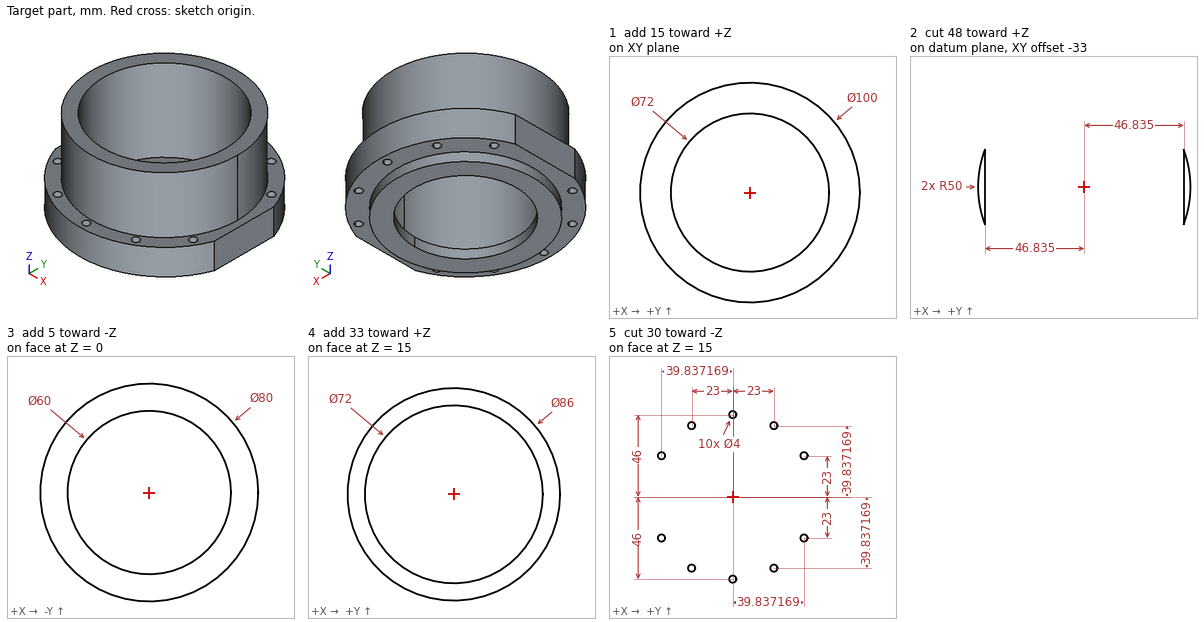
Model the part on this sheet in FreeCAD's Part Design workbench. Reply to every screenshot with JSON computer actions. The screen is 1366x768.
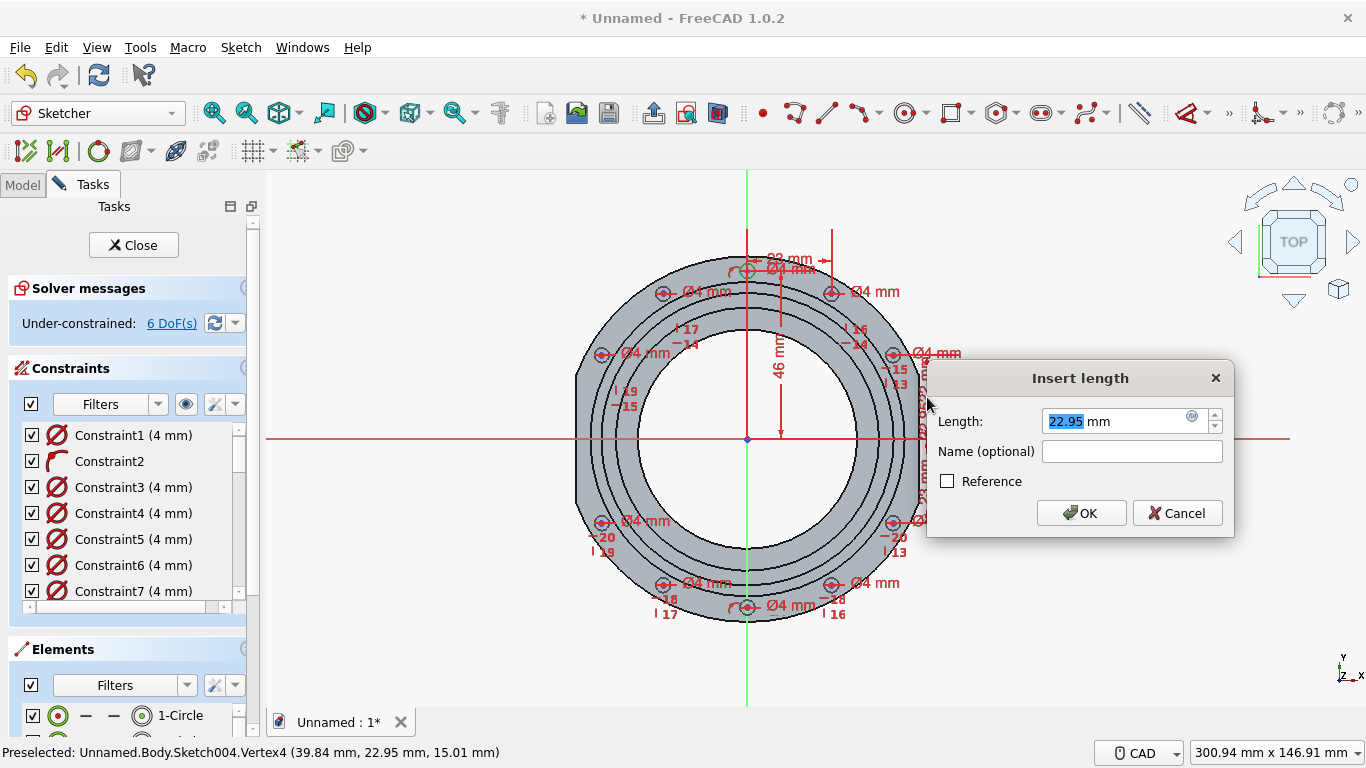
{"action": "type", "text": "23"}
{"action": "key", "text": "Return"}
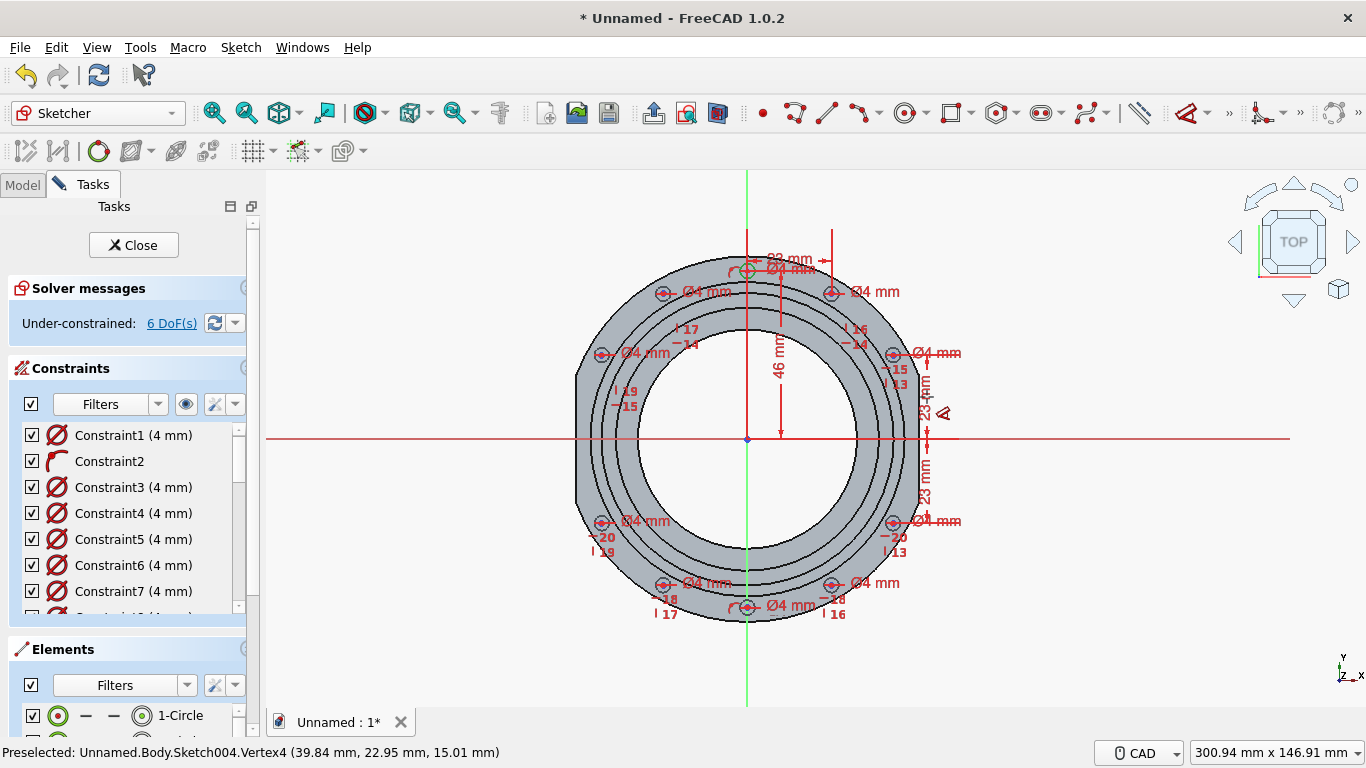
{"action": "left_click", "coordinate": [663, 294]}
{"action": "left_click", "coordinate": [705, 260]}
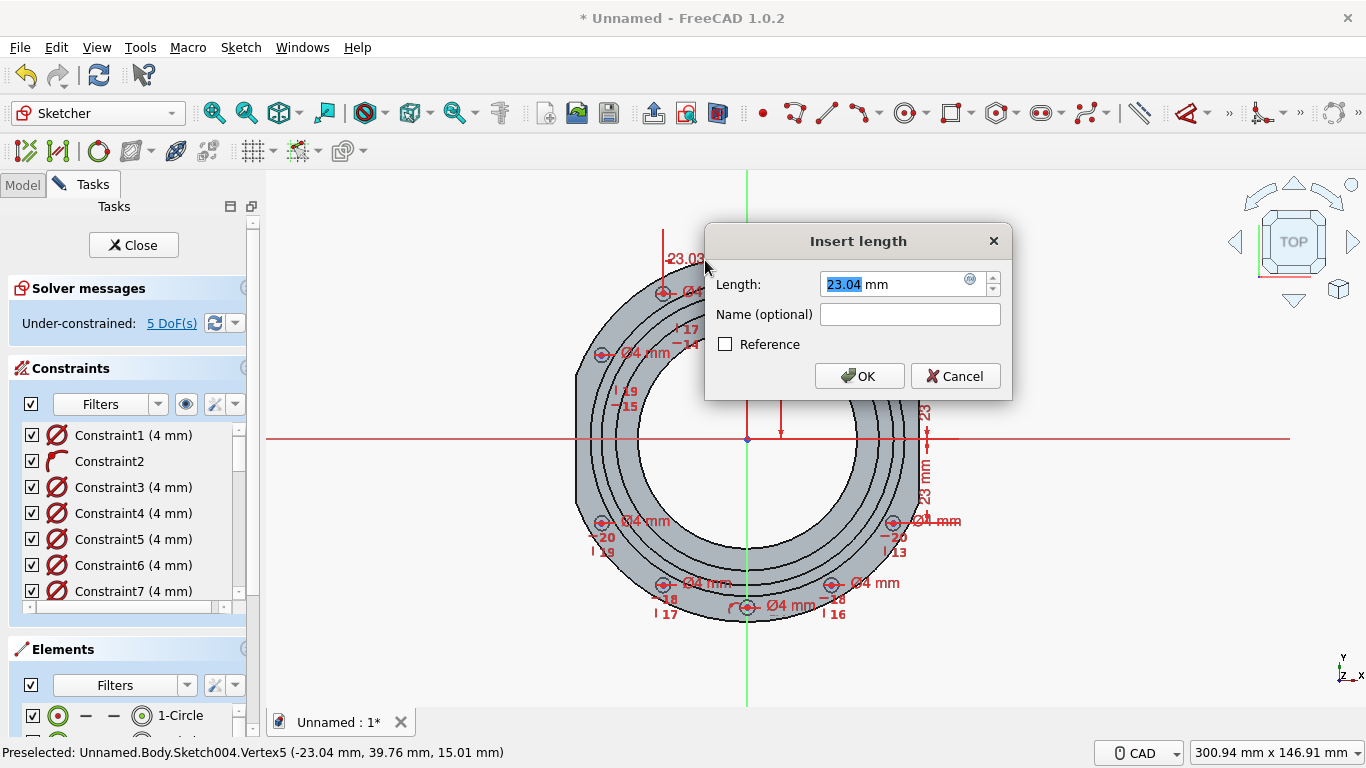
{"action": "type", "text": "23"}
{"action": "key", "text": "Return"}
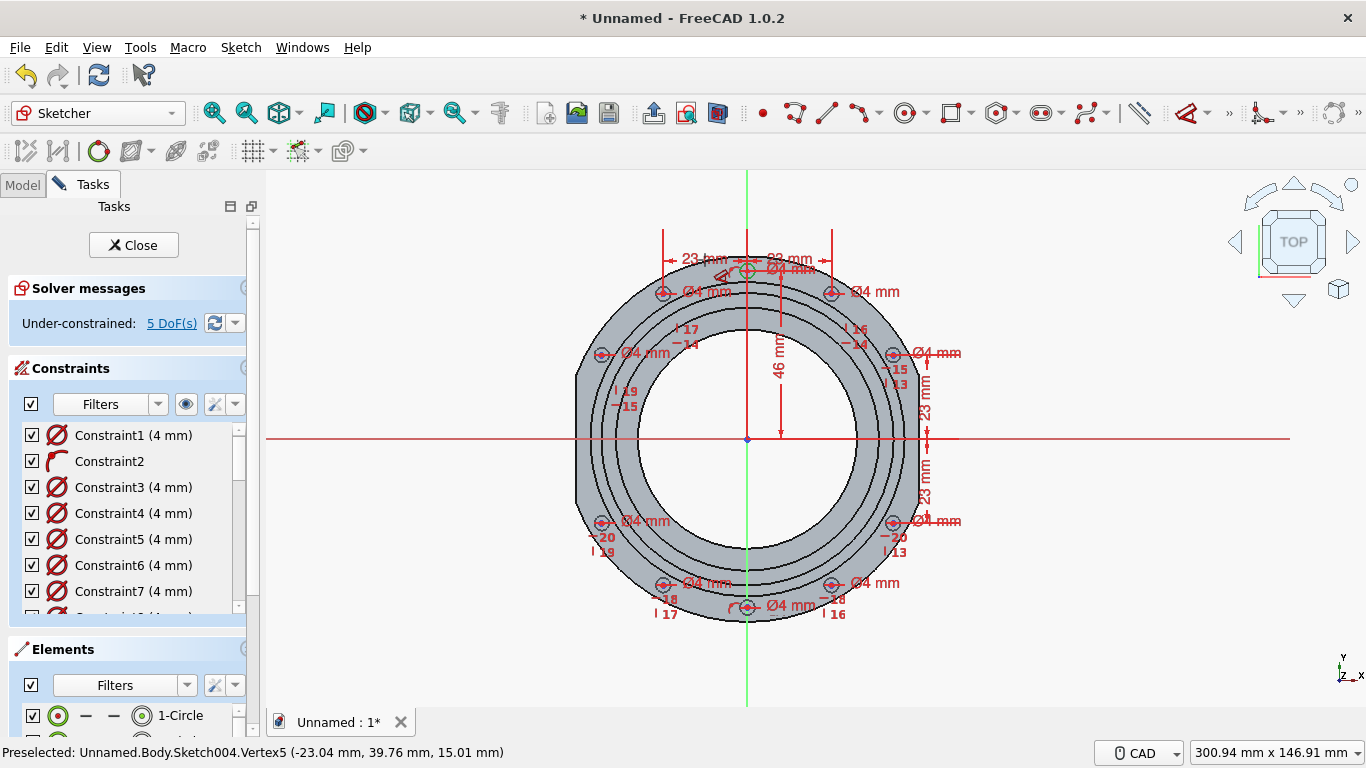
{"action": "left_click", "coordinate": [747, 608]}
{"action": "left_click", "coordinate": [781, 523]}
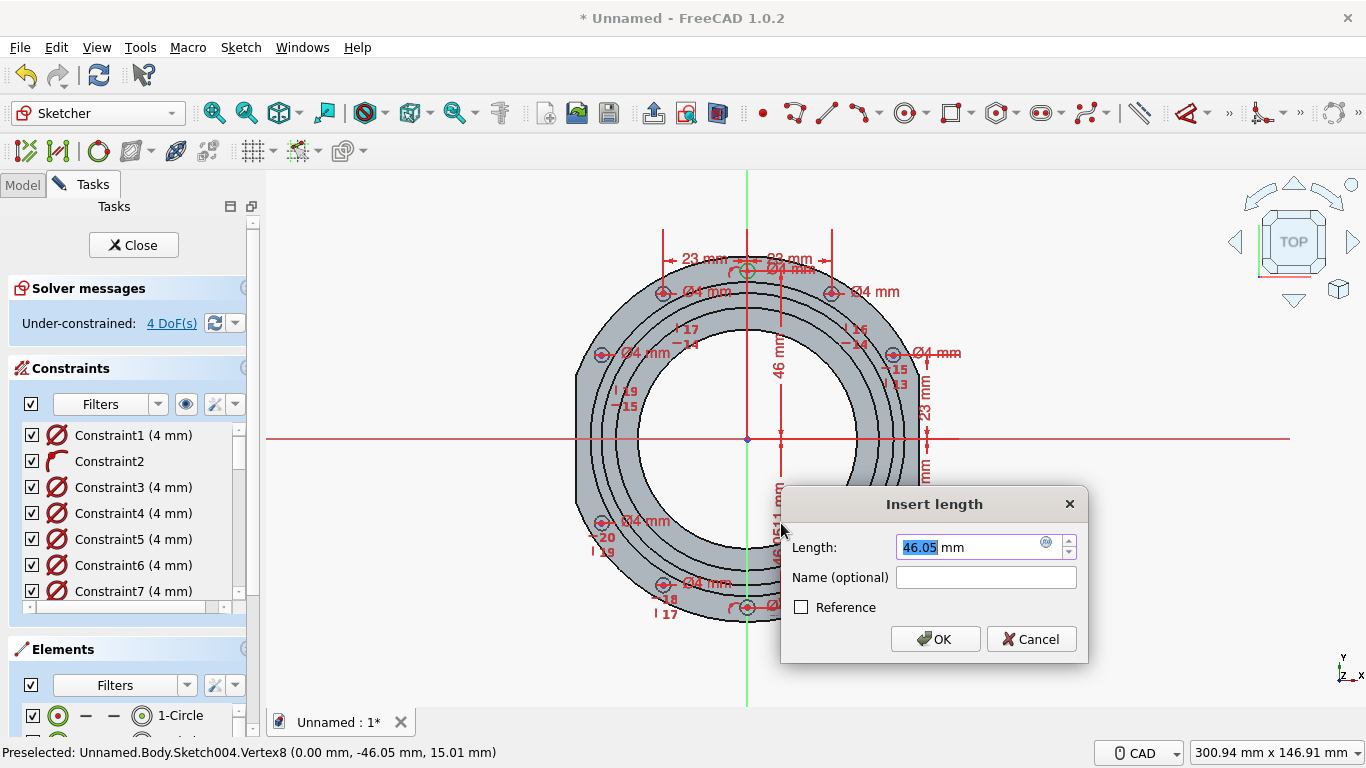
{"action": "type", "text": "46"}
{"action": "key", "text": "Return"}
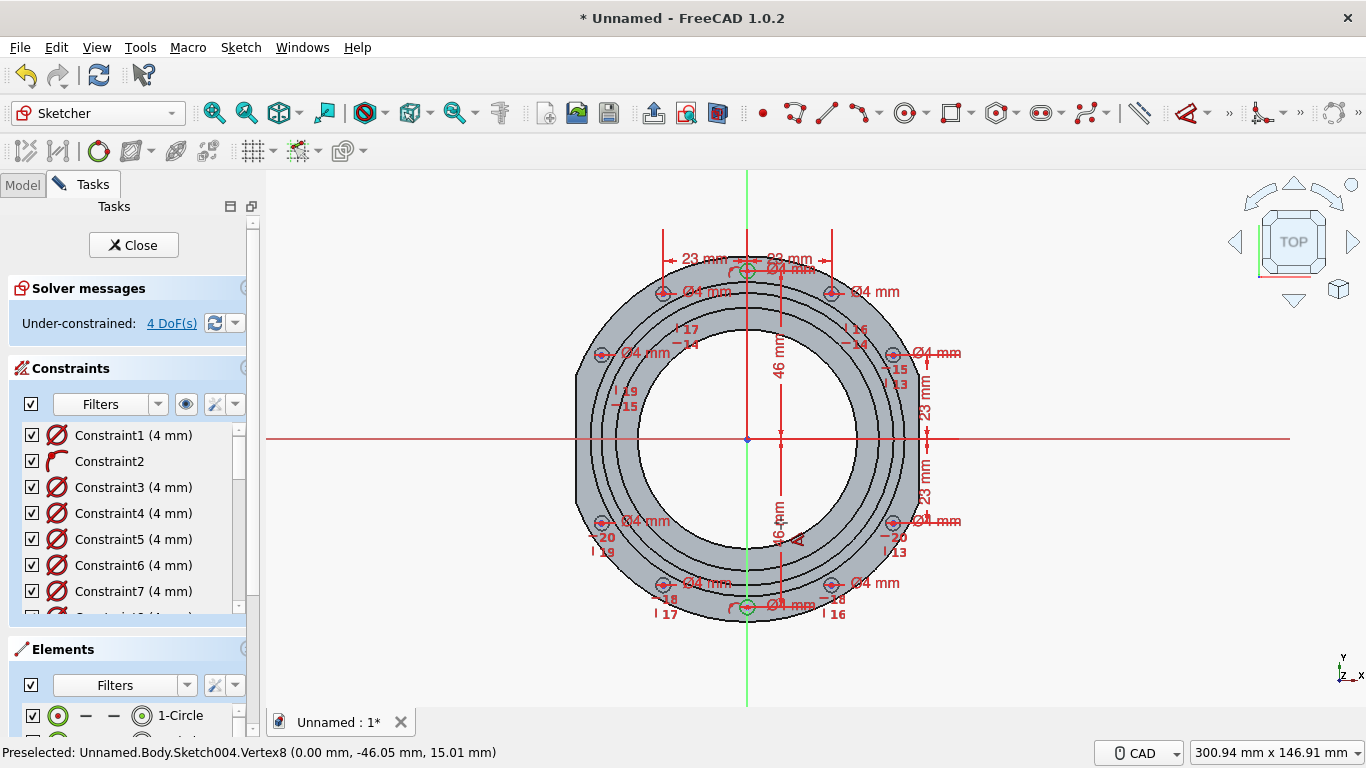
{"action": "left_click", "coordinate": [893, 523]}
{"action": "left_click", "coordinate": [820, 557]}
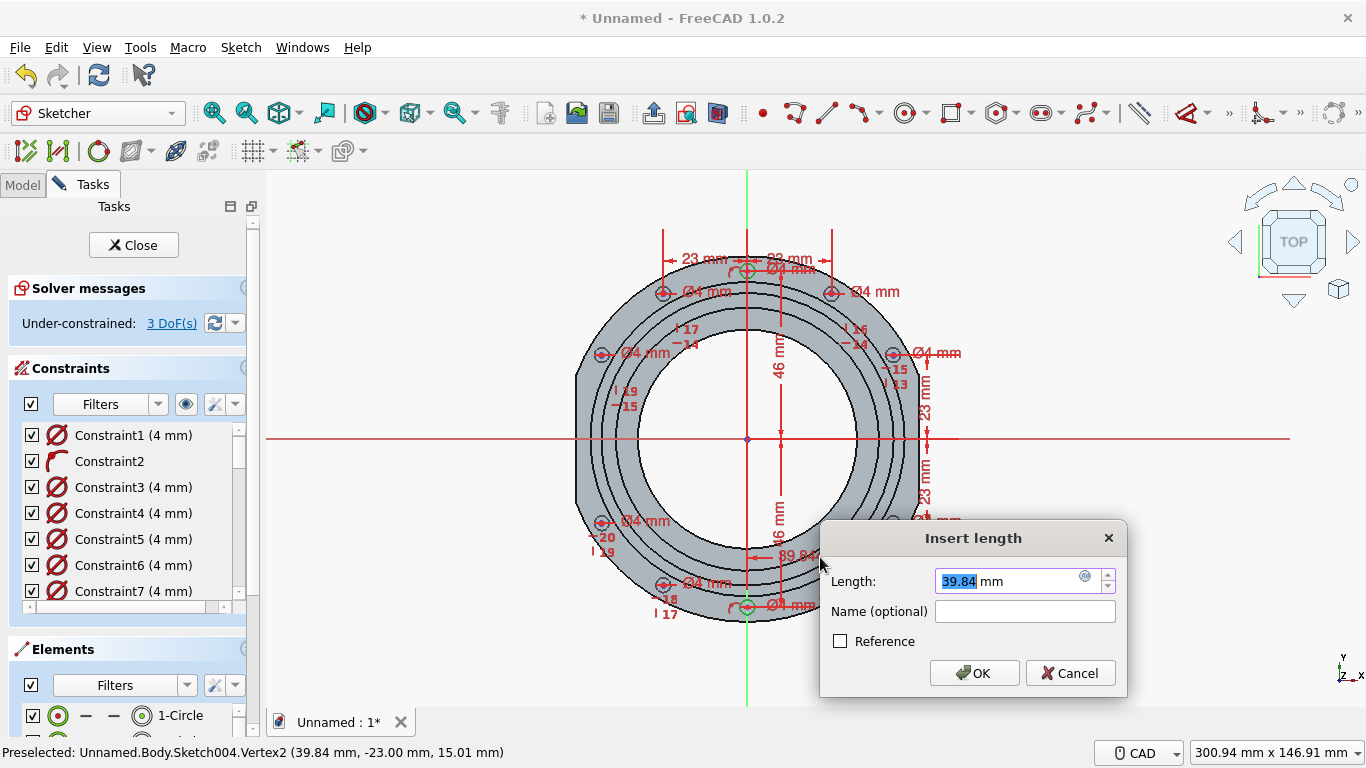
{"action": "type", "text": "39.837169"}
{"action": "key", "text": "Return"}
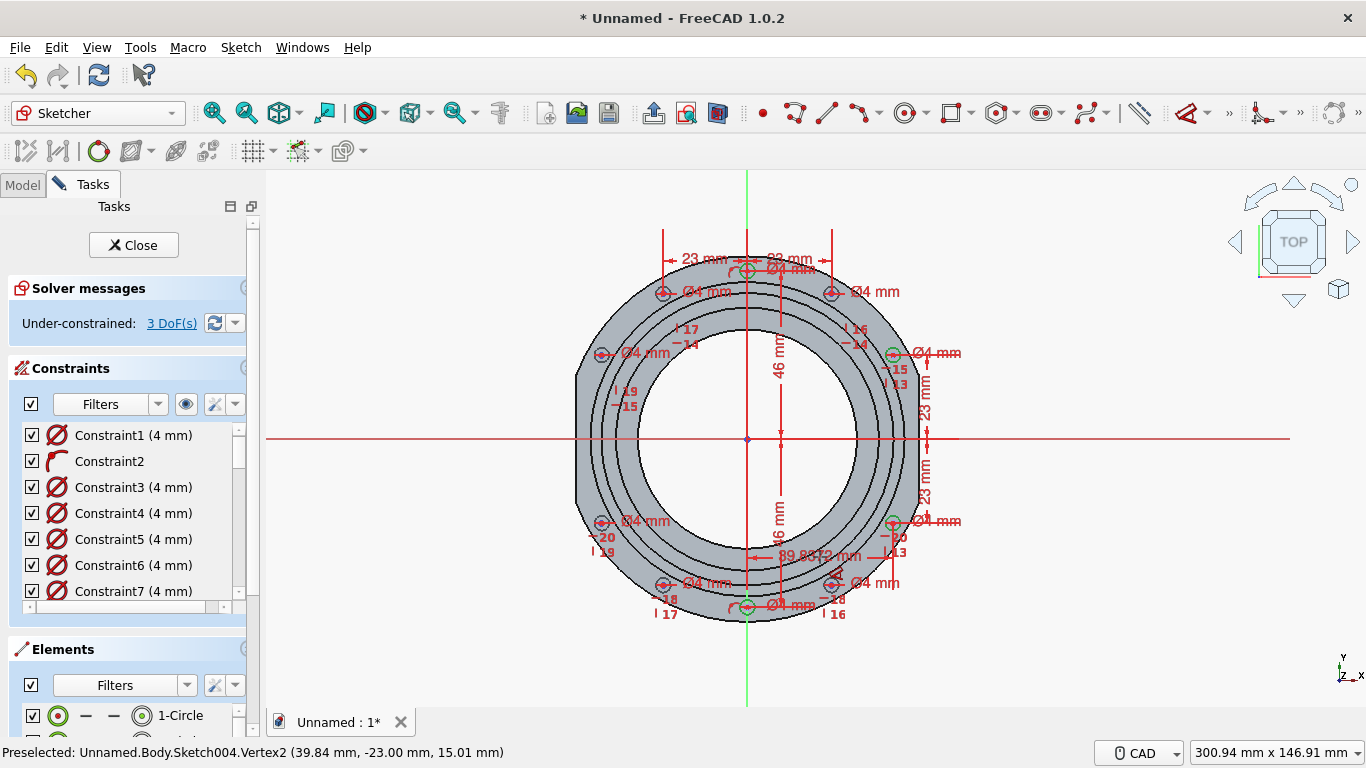
{"action": "left_click", "coordinate": [832, 294]}
{"action": "left_click", "coordinate": [866, 367]}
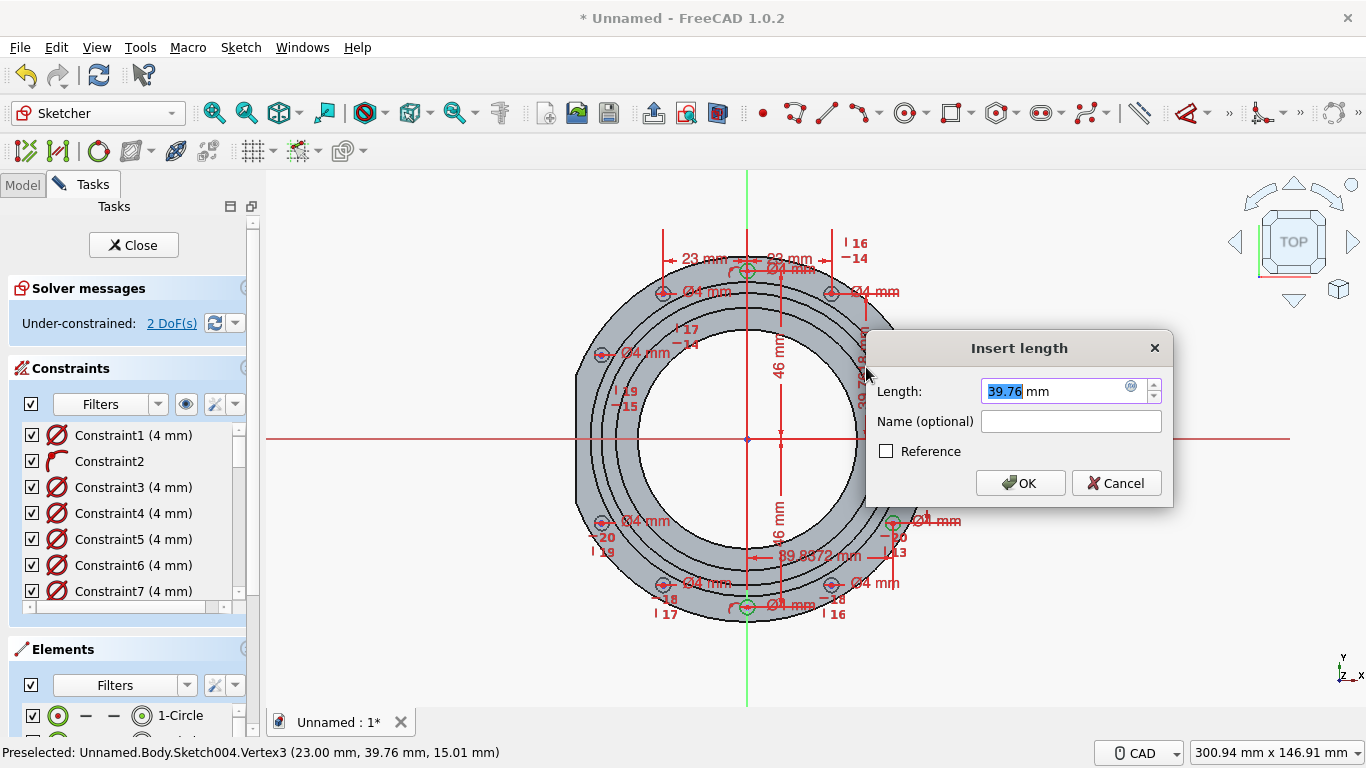
{"action": "type", "text": "39.837169"}
{"action": "key", "text": "Return"}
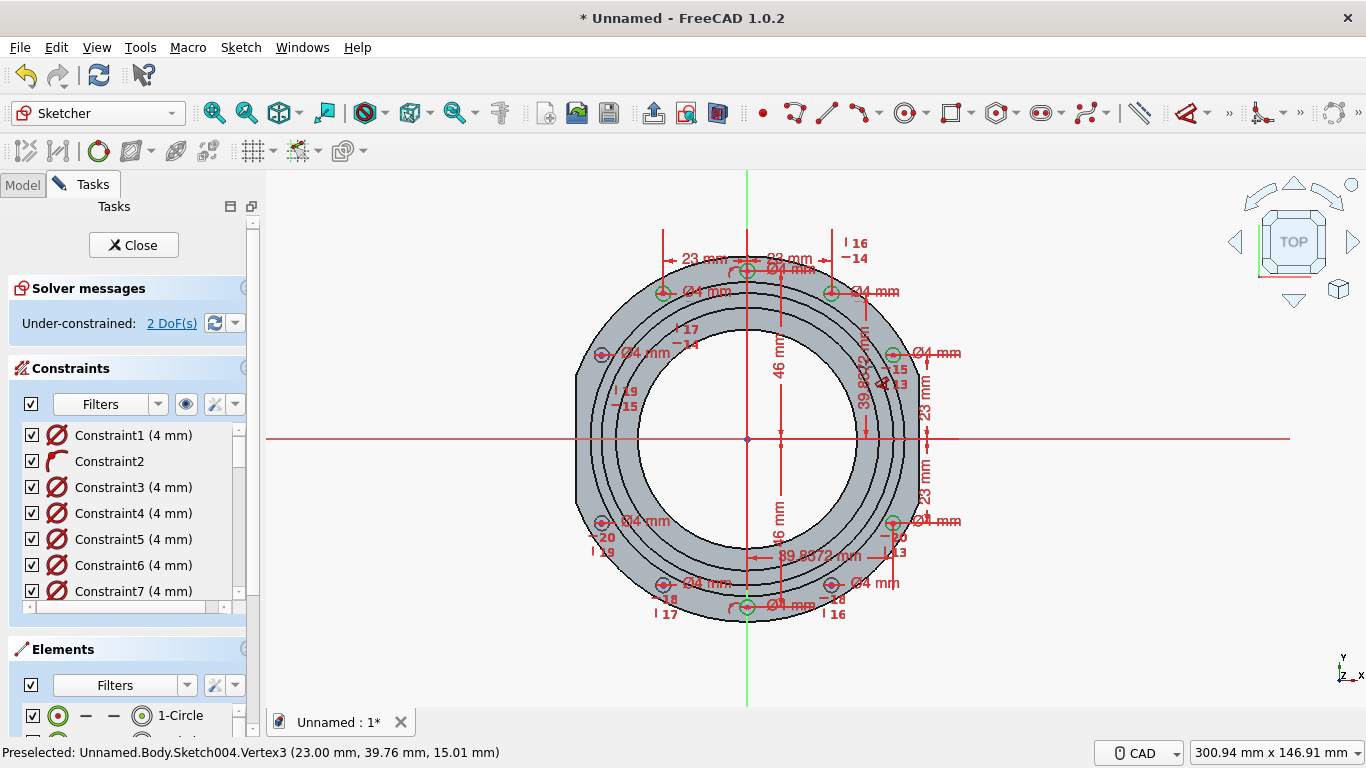
{"action": "left_click", "coordinate": [602, 355]}
{"action": "left_click", "coordinate": [675, 321]}